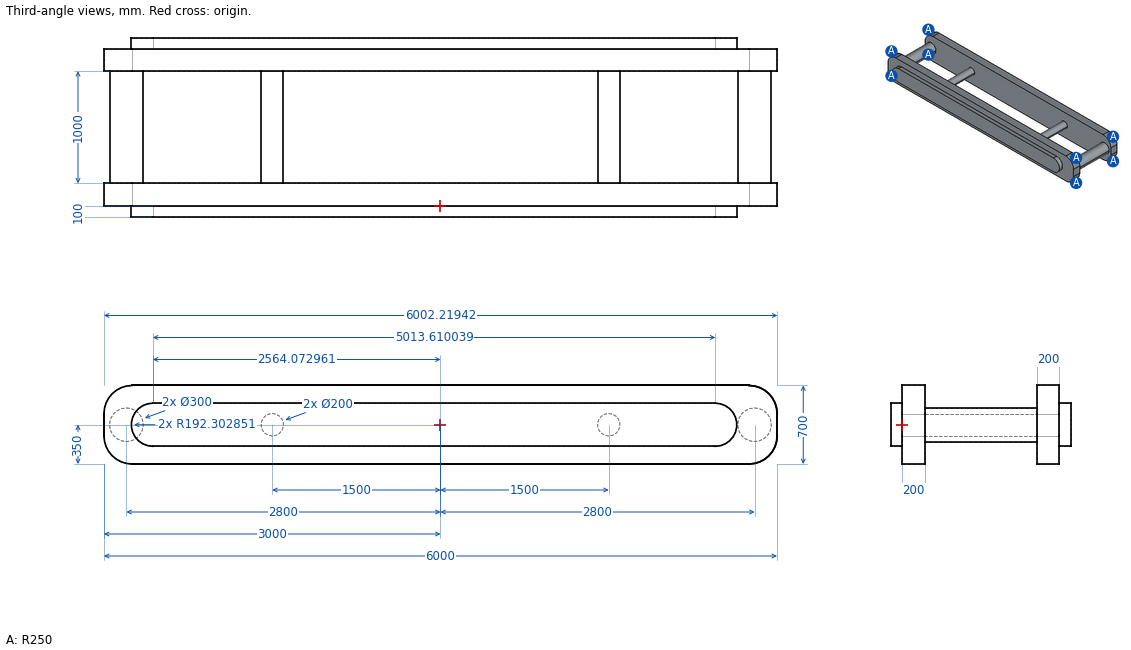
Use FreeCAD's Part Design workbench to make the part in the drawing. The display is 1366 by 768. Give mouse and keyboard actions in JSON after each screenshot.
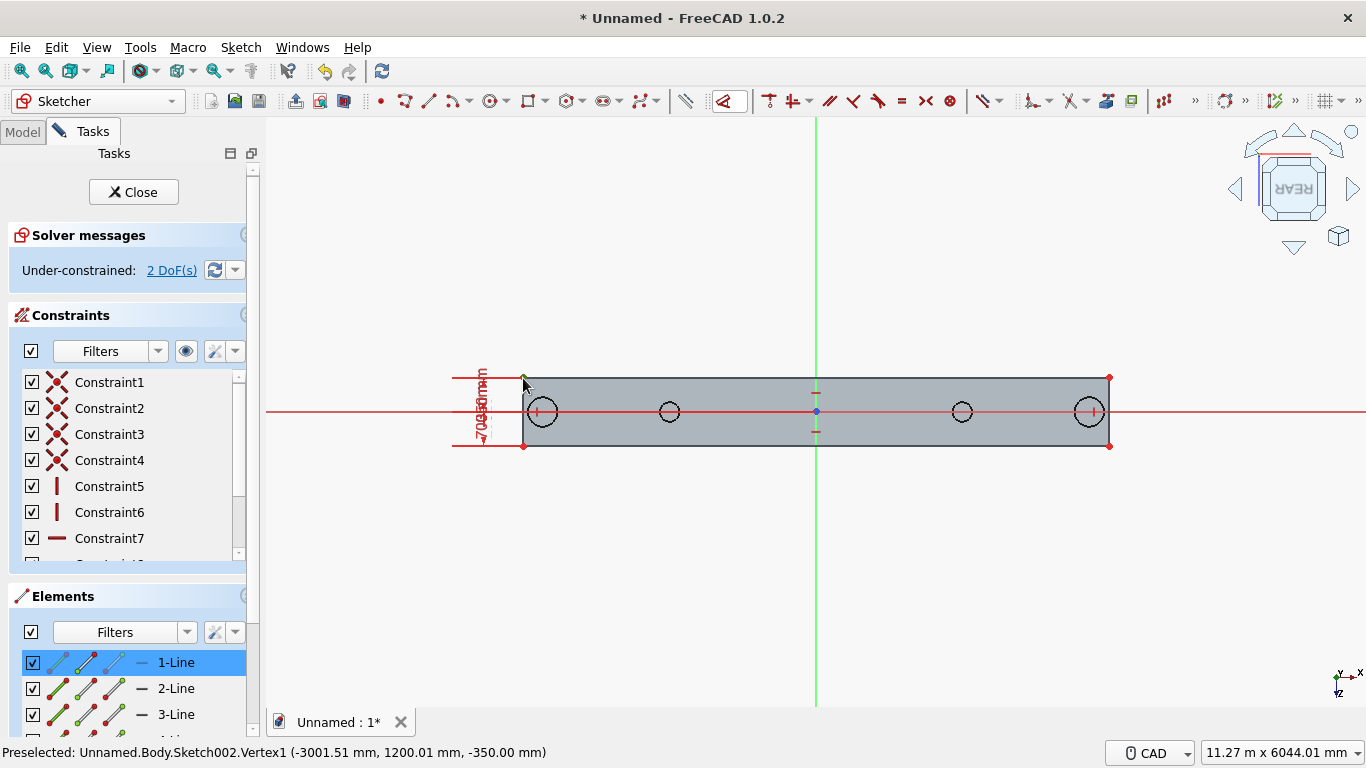
{"action": "left_click", "coordinate": [742, 102]}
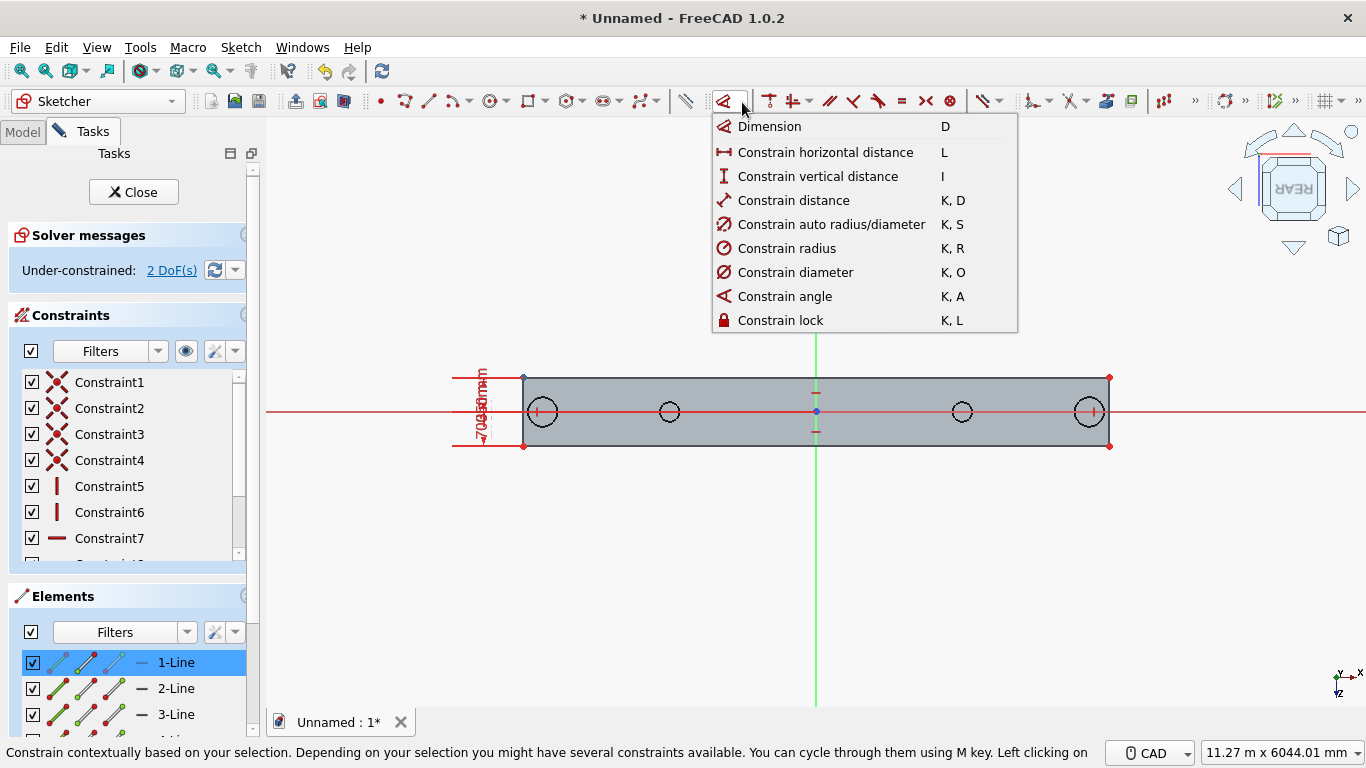
{"action": "left_click", "coordinate": [865, 152]}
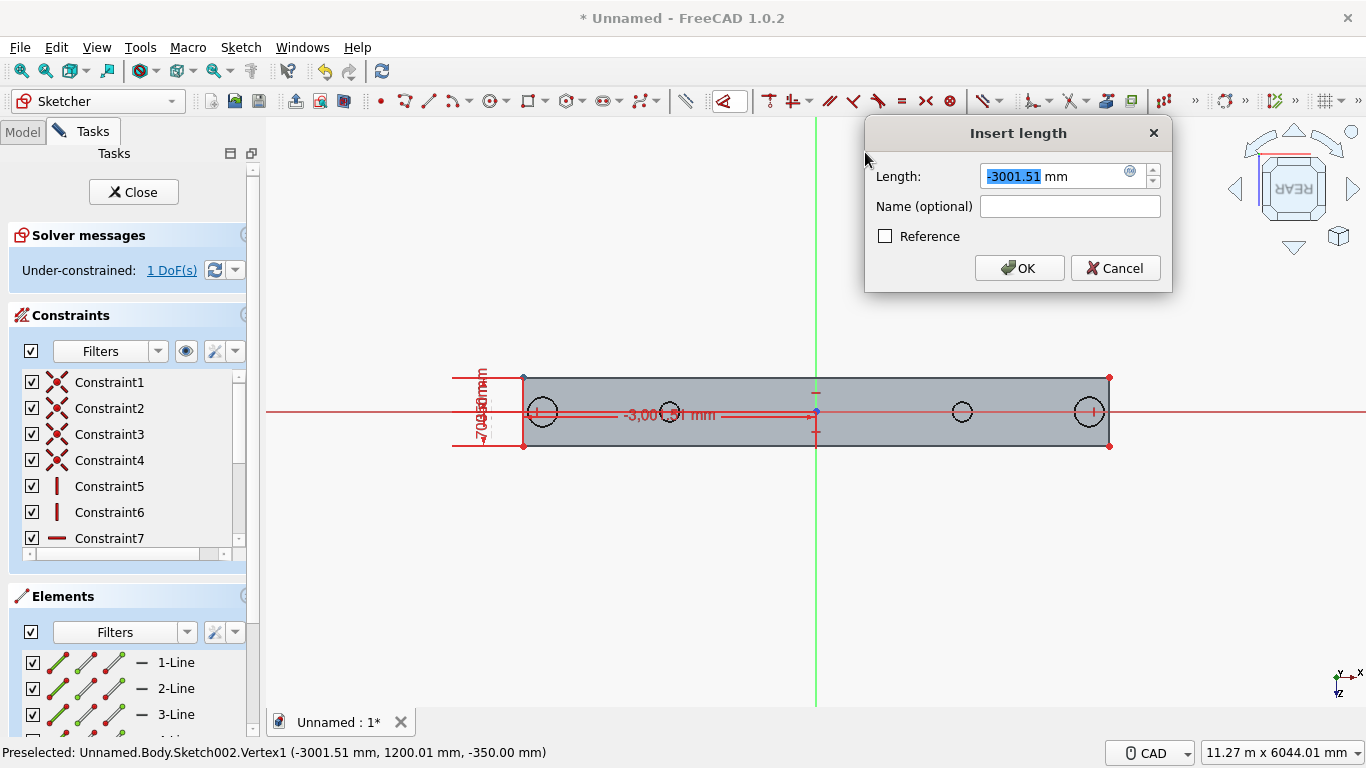
{"action": "type", "text": "-3000"}
{"action": "key", "text": "Return"}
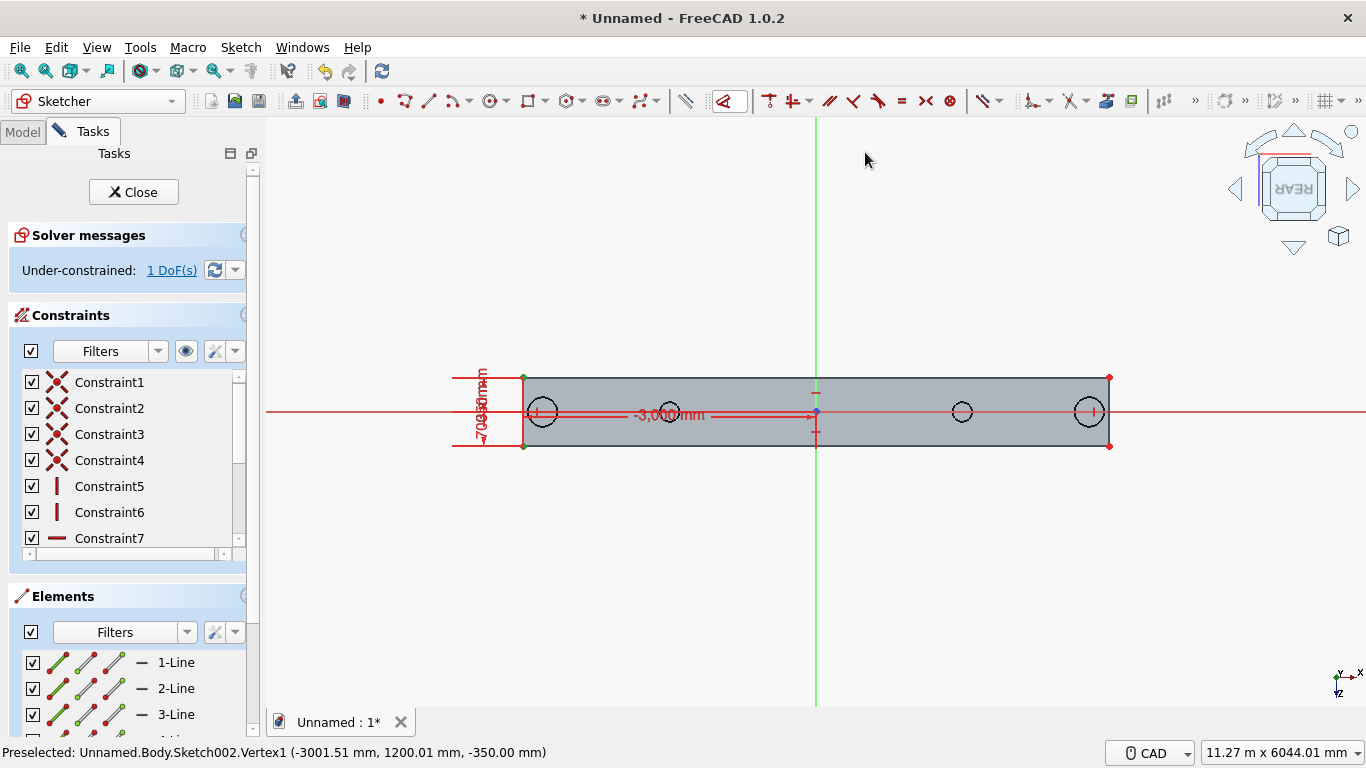
{"action": "left_click", "coordinate": [699, 446]}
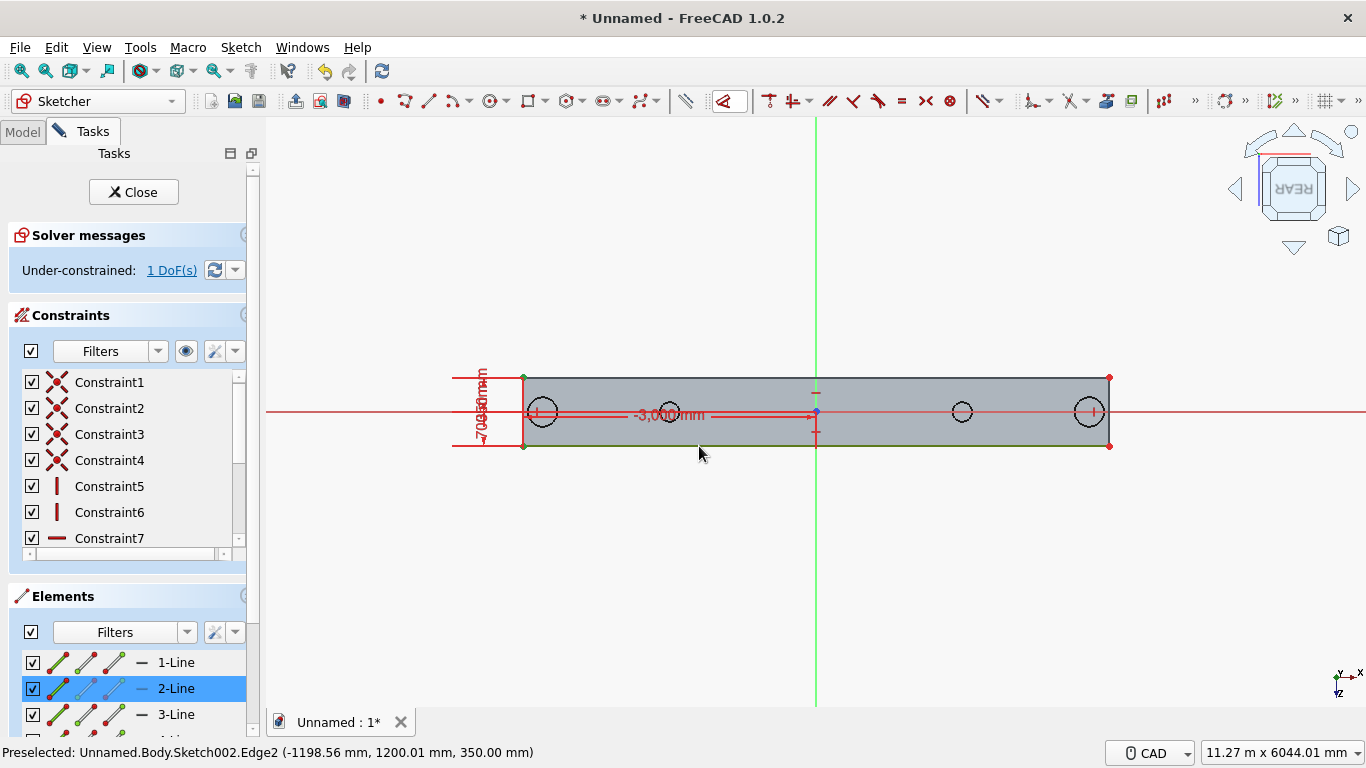
{"action": "key", "text": "l"}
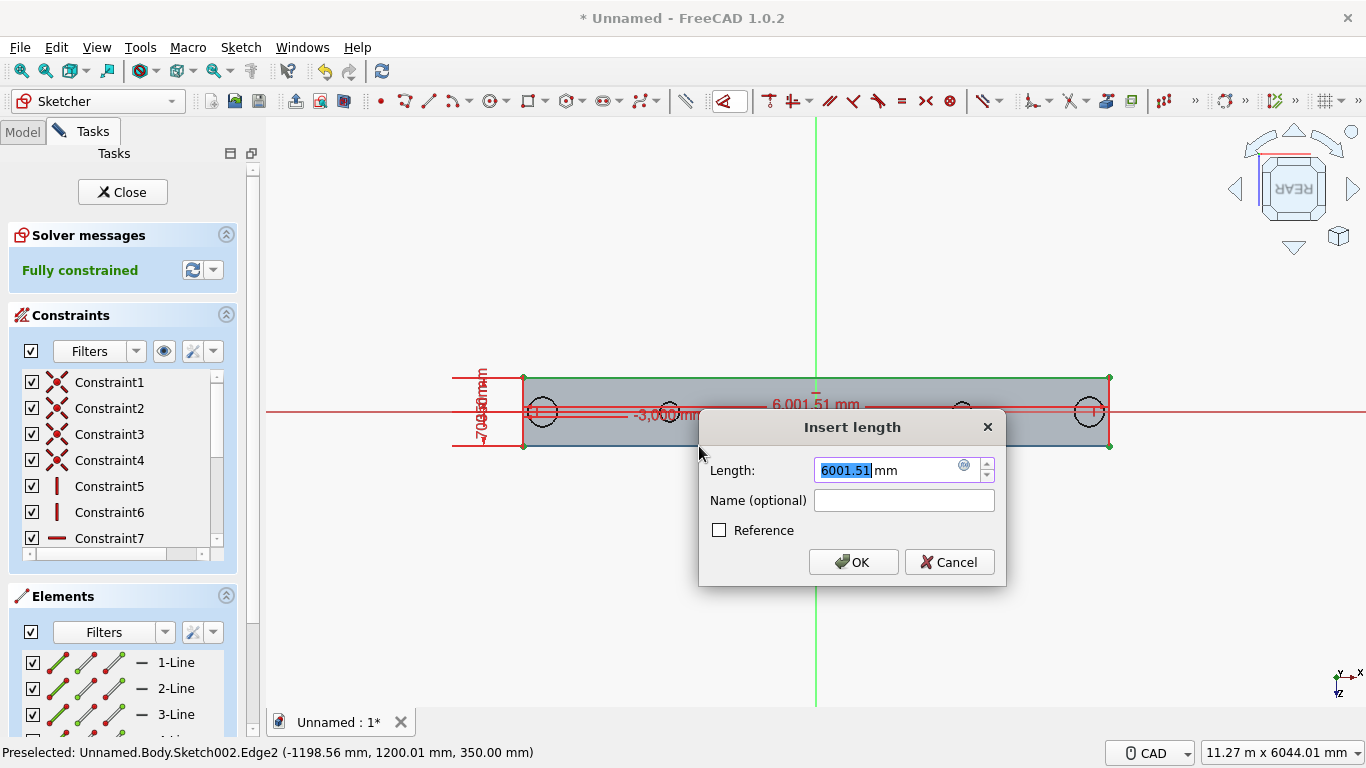
{"action": "type", "text": "6002.21942"}
{"action": "key", "text": "Return"}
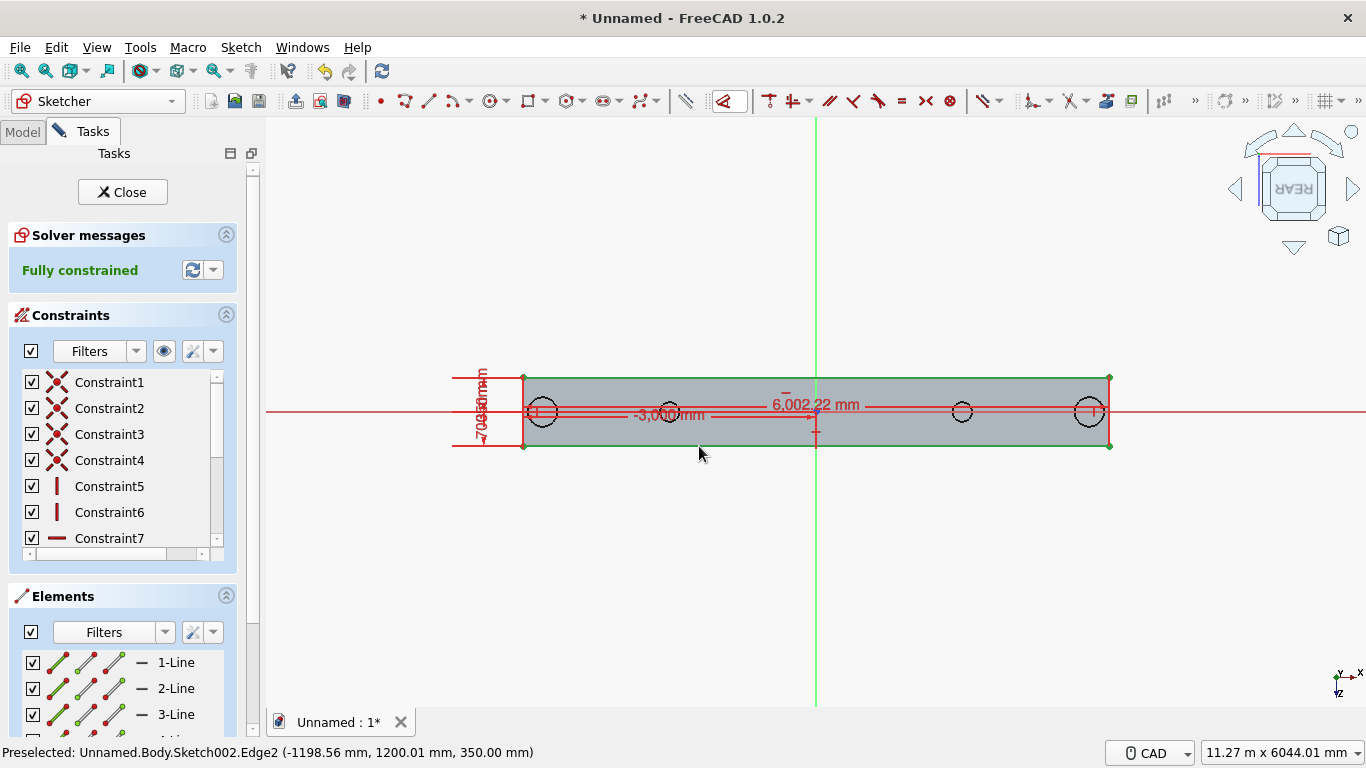
{"action": "left_click", "coordinate": [123, 192]}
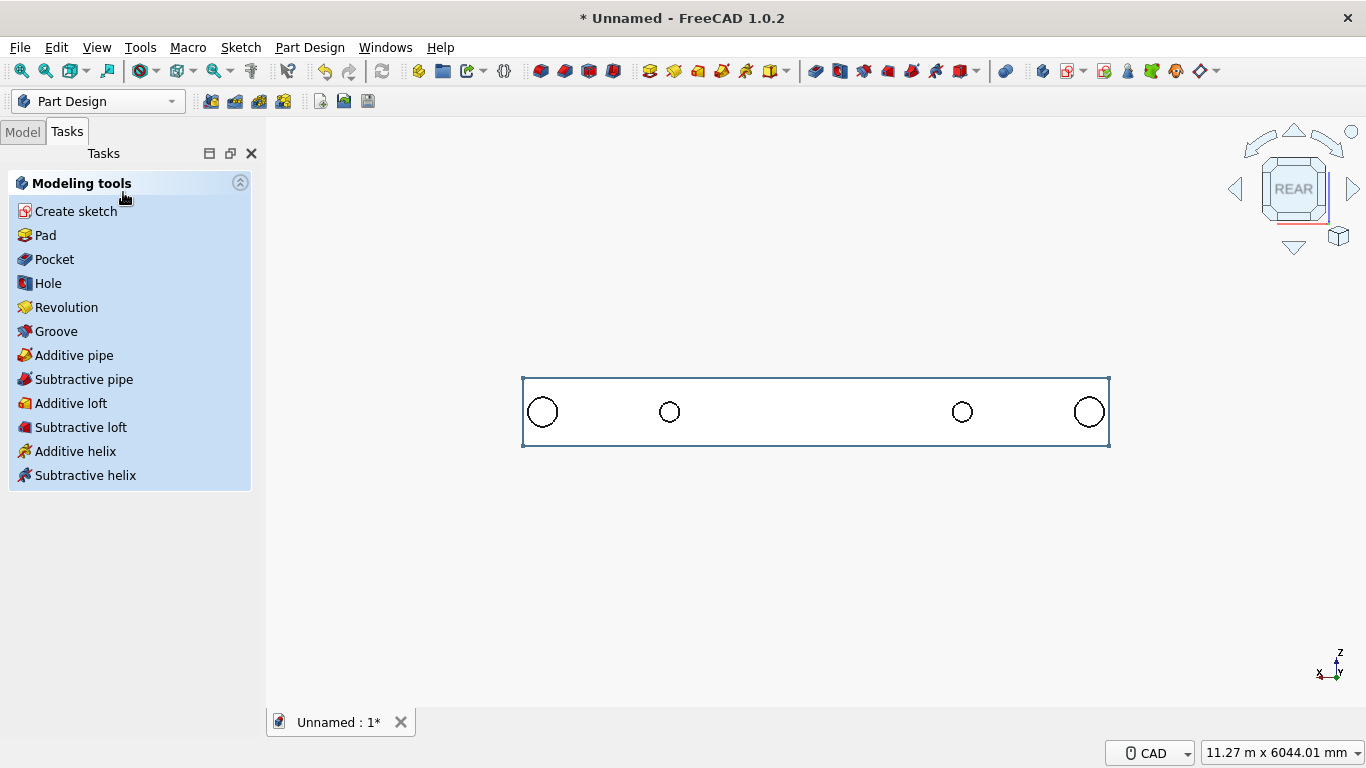
{"action": "left_click", "coordinate": [650, 72]}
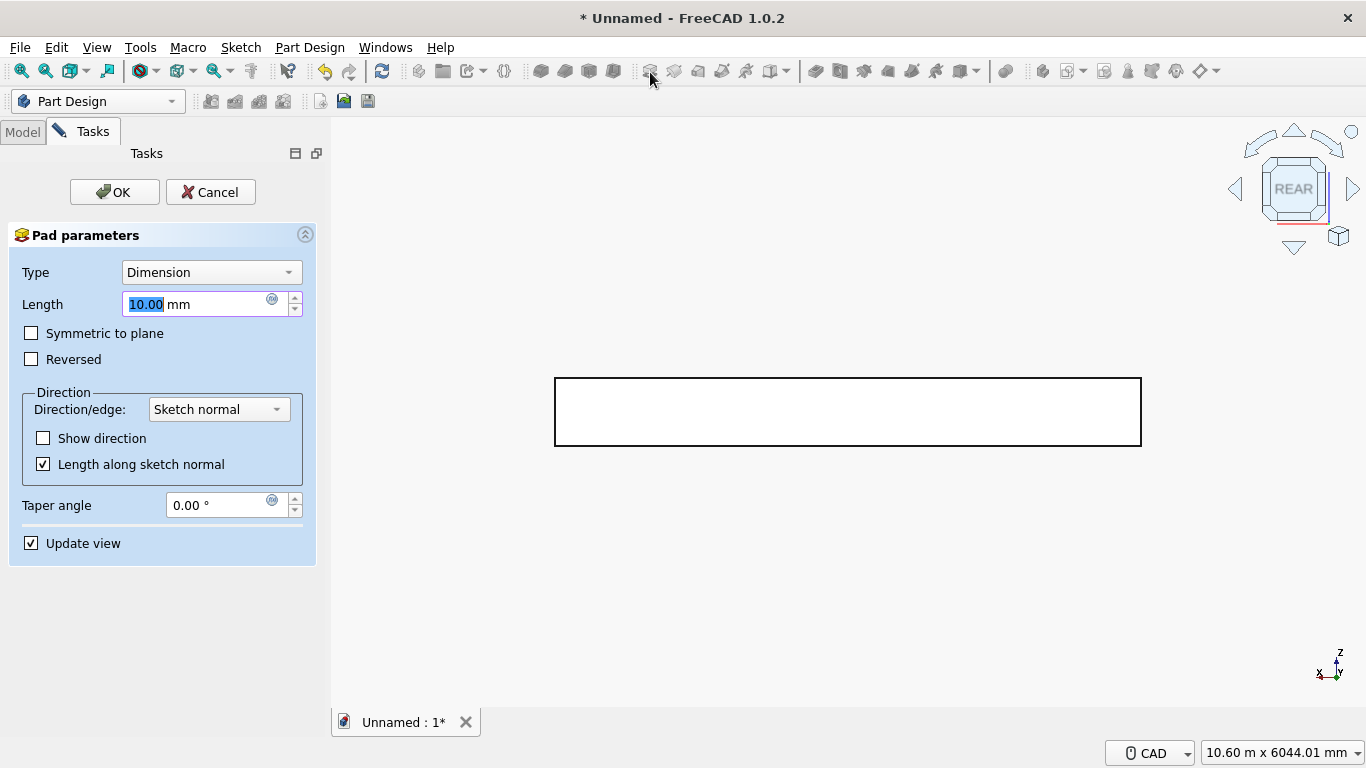
{"action": "type", "text": "200"}
{"action": "key", "text": "Tab"}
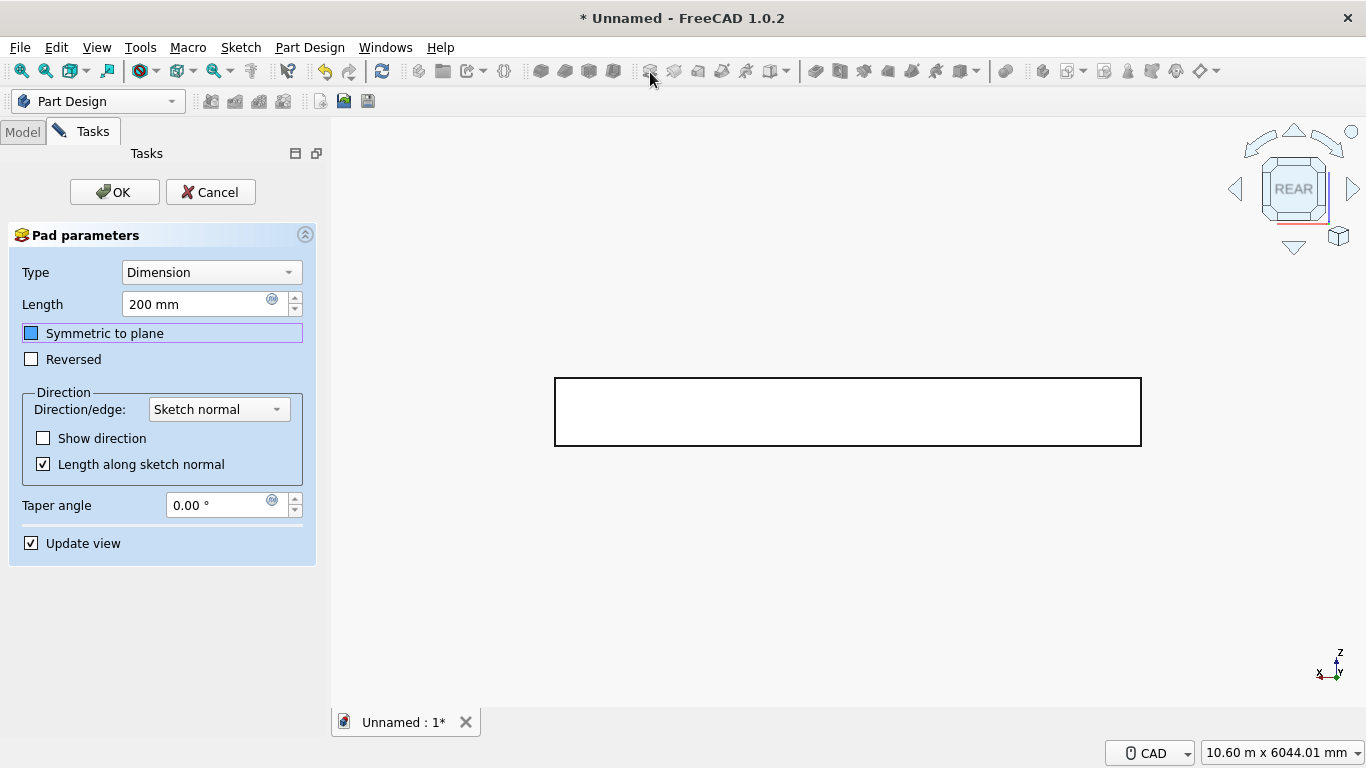
{"action": "left_click", "coordinate": [115, 192]}